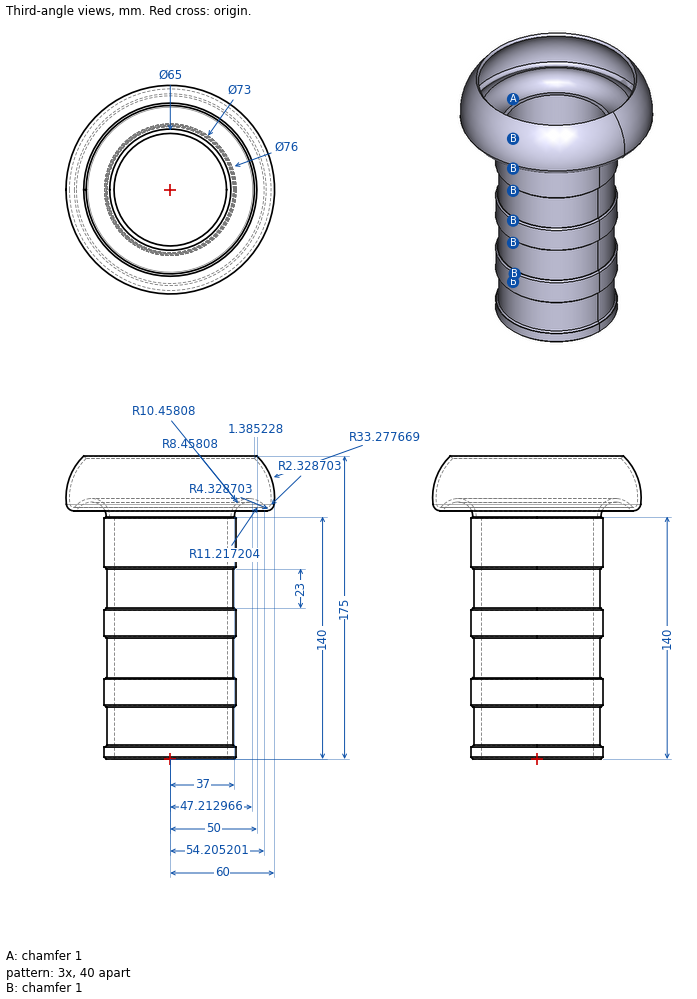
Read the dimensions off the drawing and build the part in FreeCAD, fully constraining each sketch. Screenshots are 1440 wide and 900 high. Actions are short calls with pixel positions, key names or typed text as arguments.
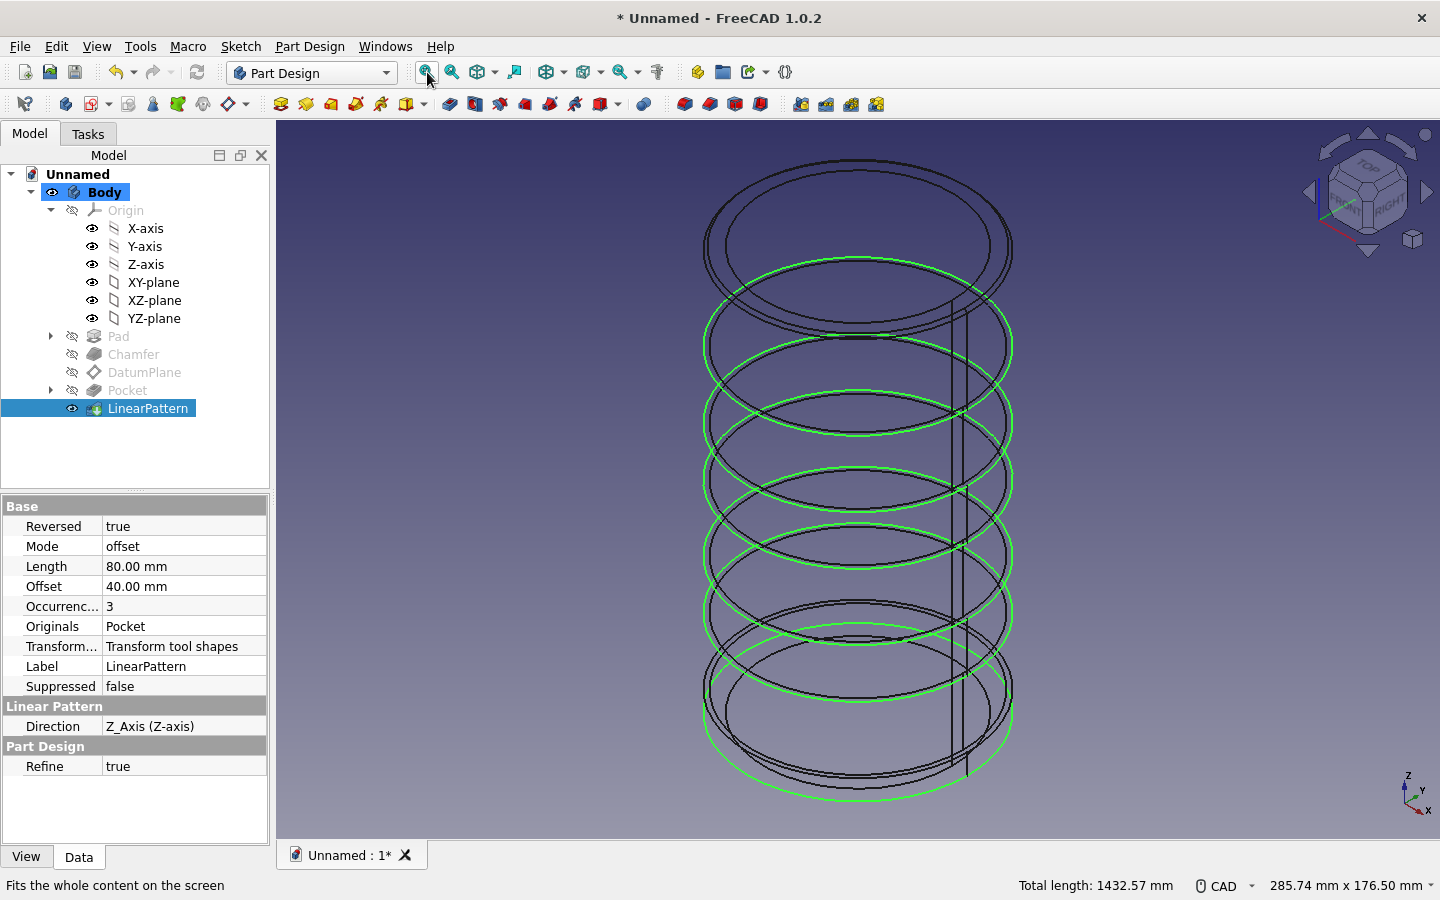
click(835, 603, ctrl)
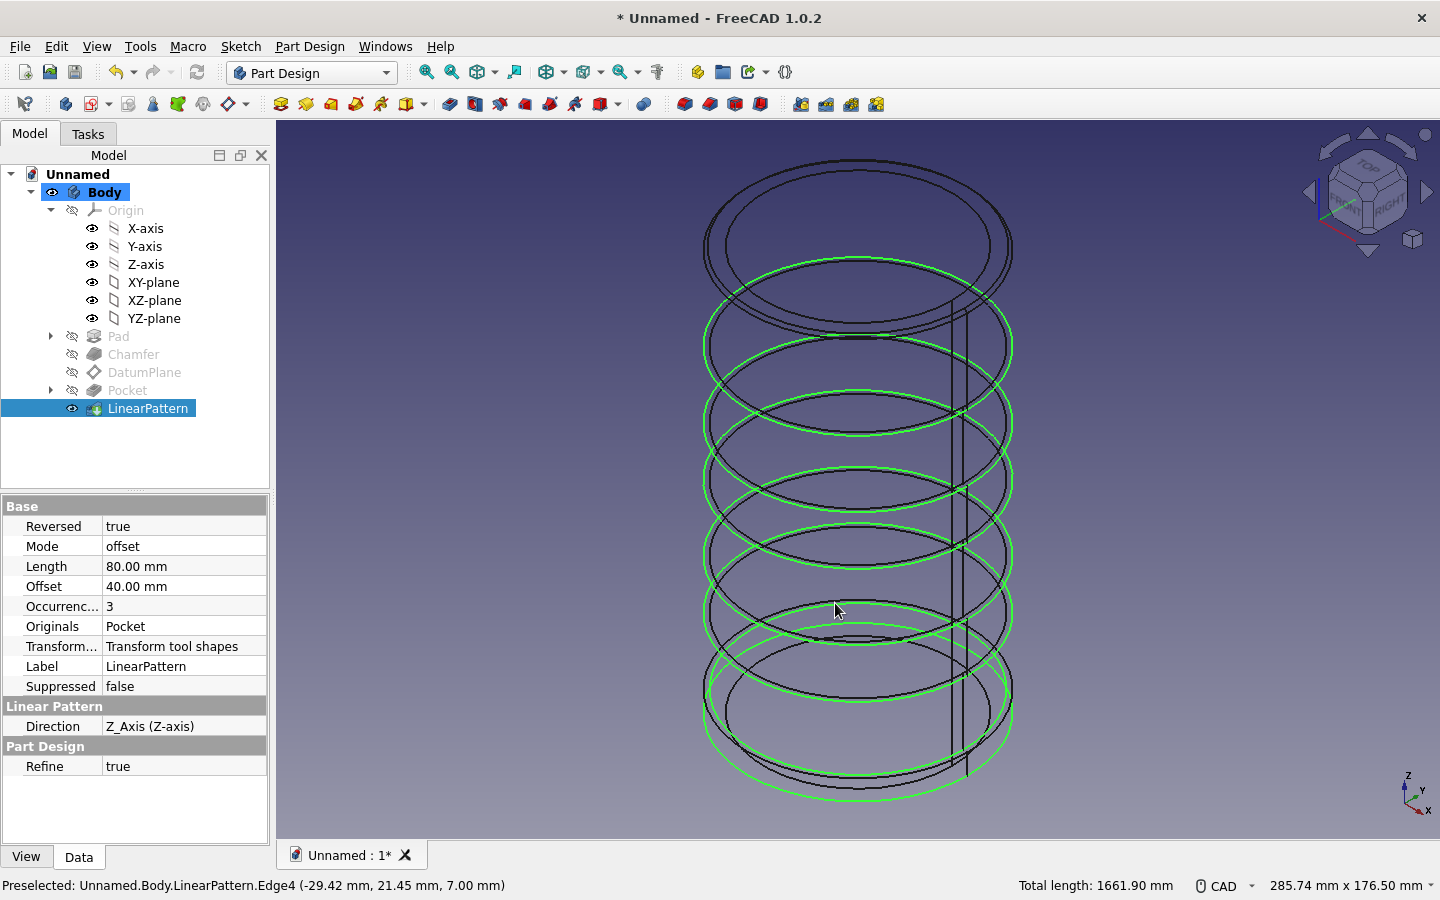
key(v)
key(1)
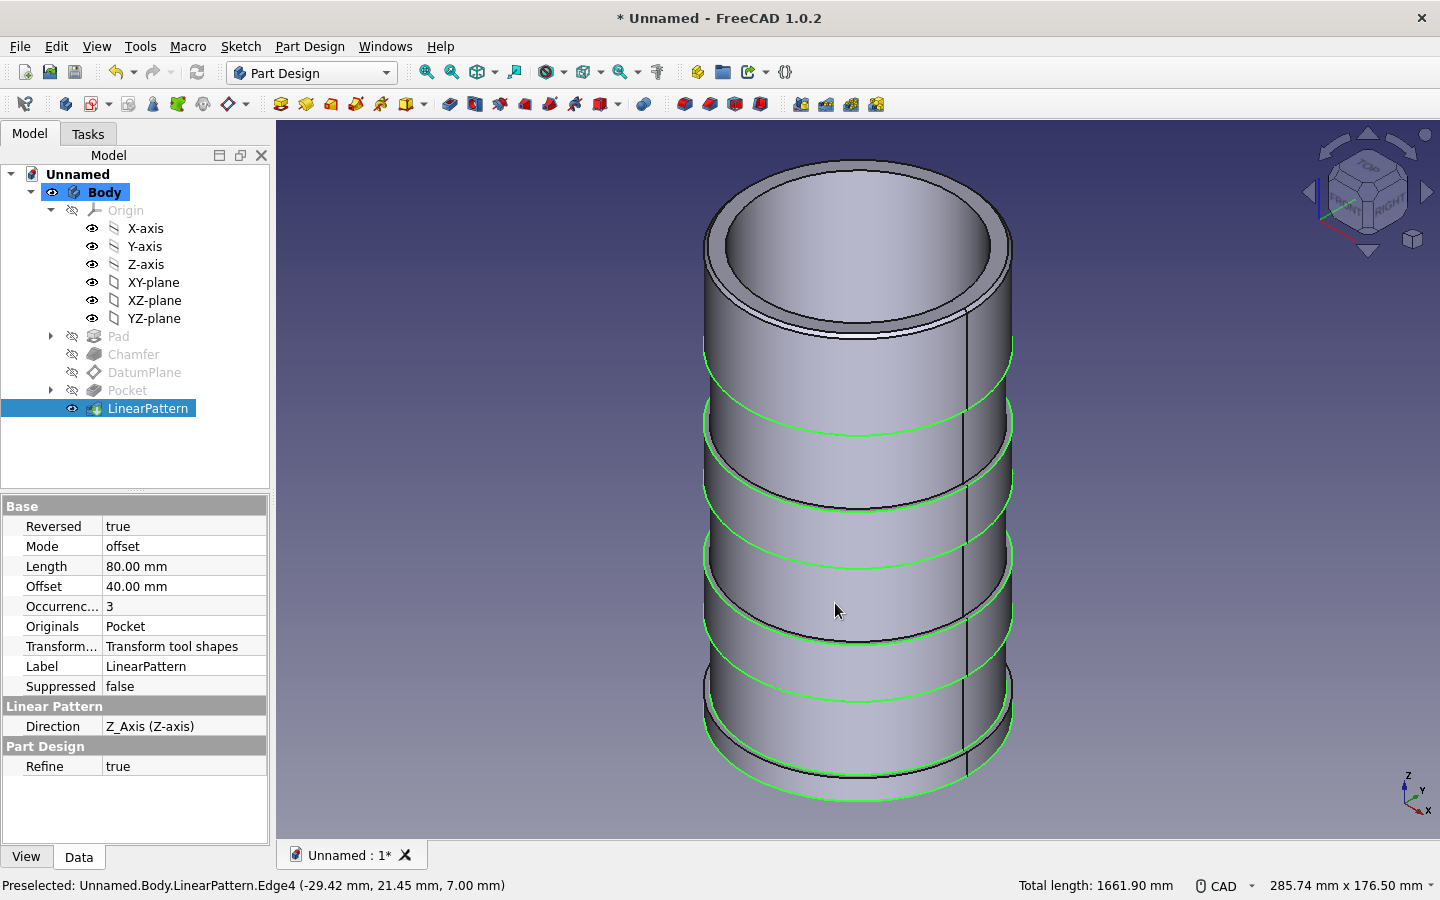
click(710, 104)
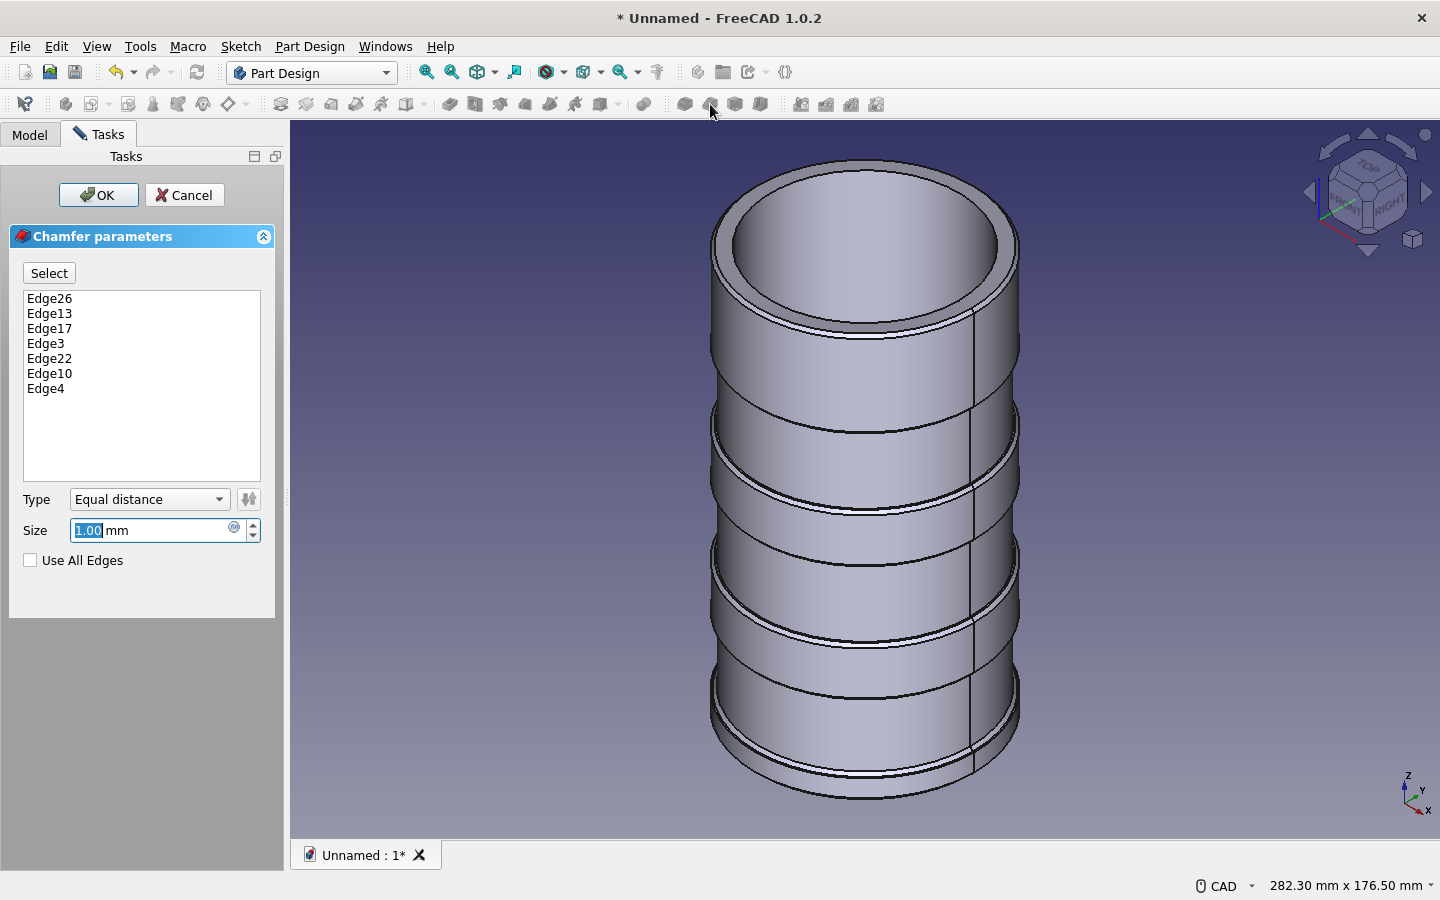
text(1)
key(Tab)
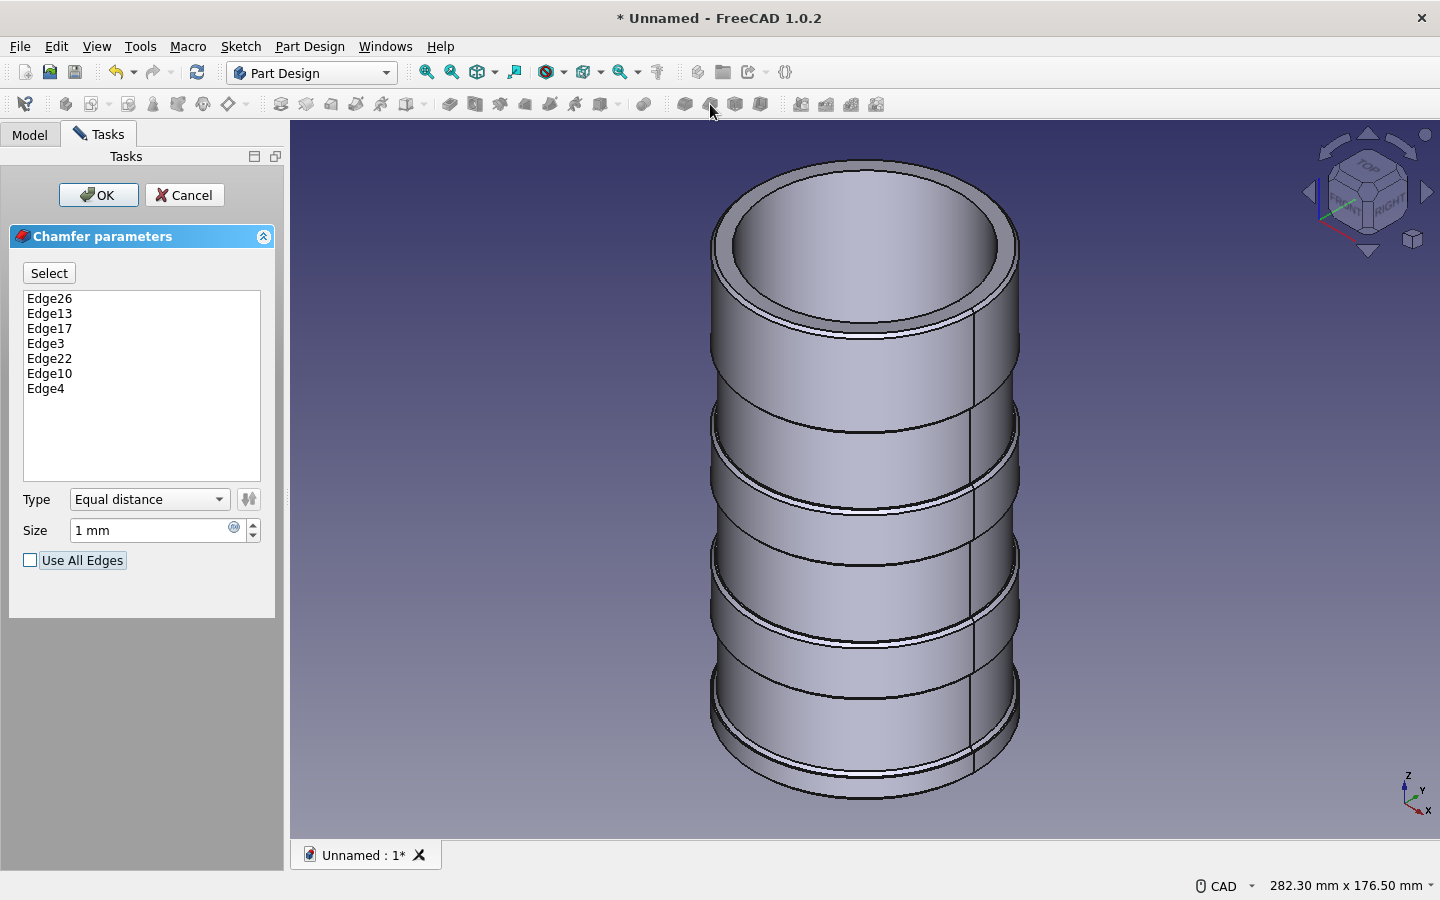
click(99, 195)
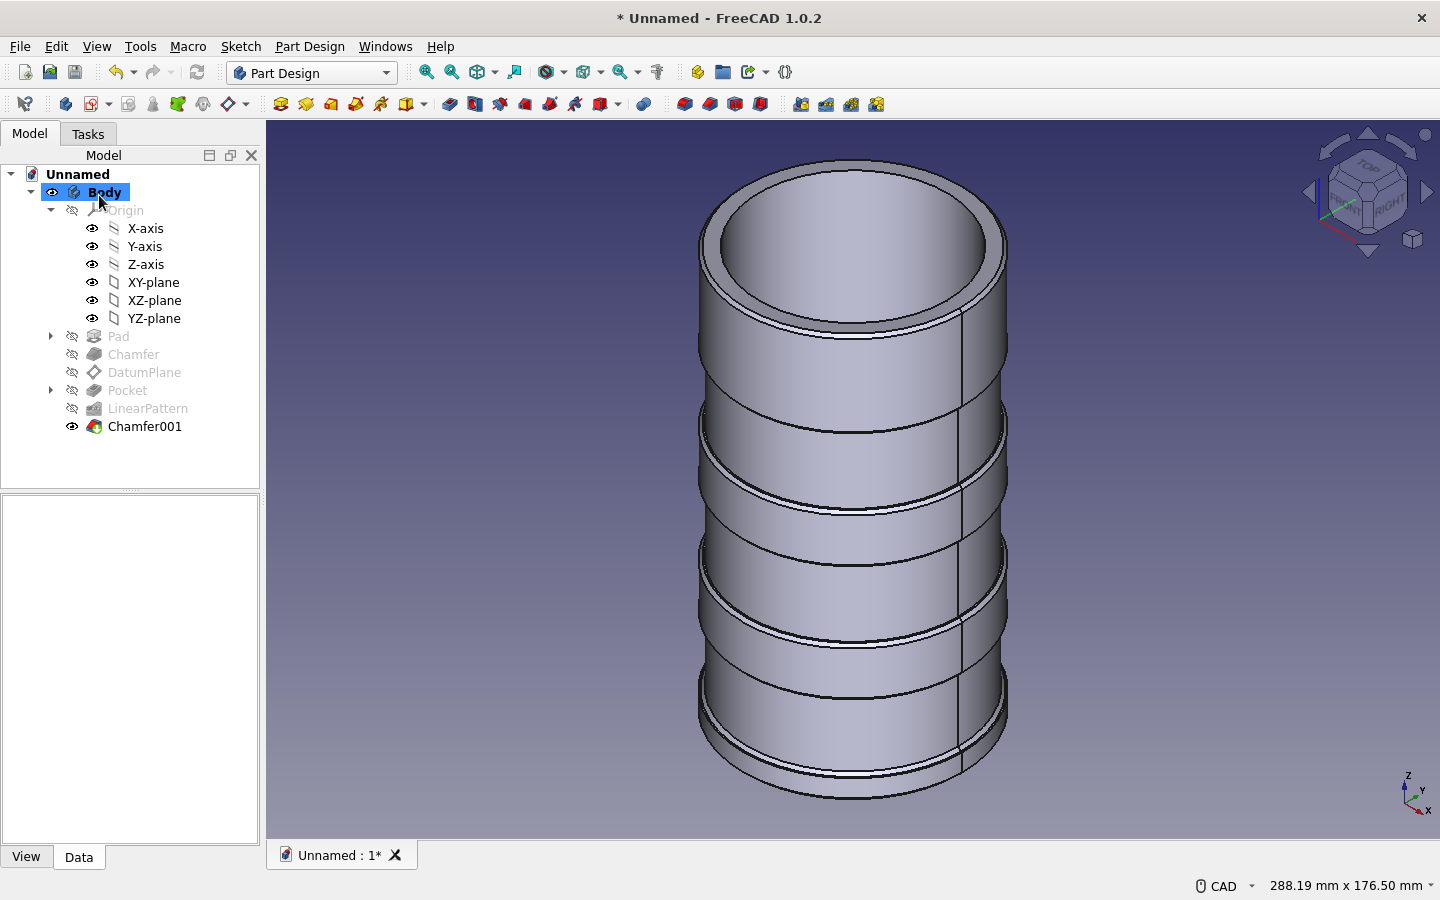
click(427, 72)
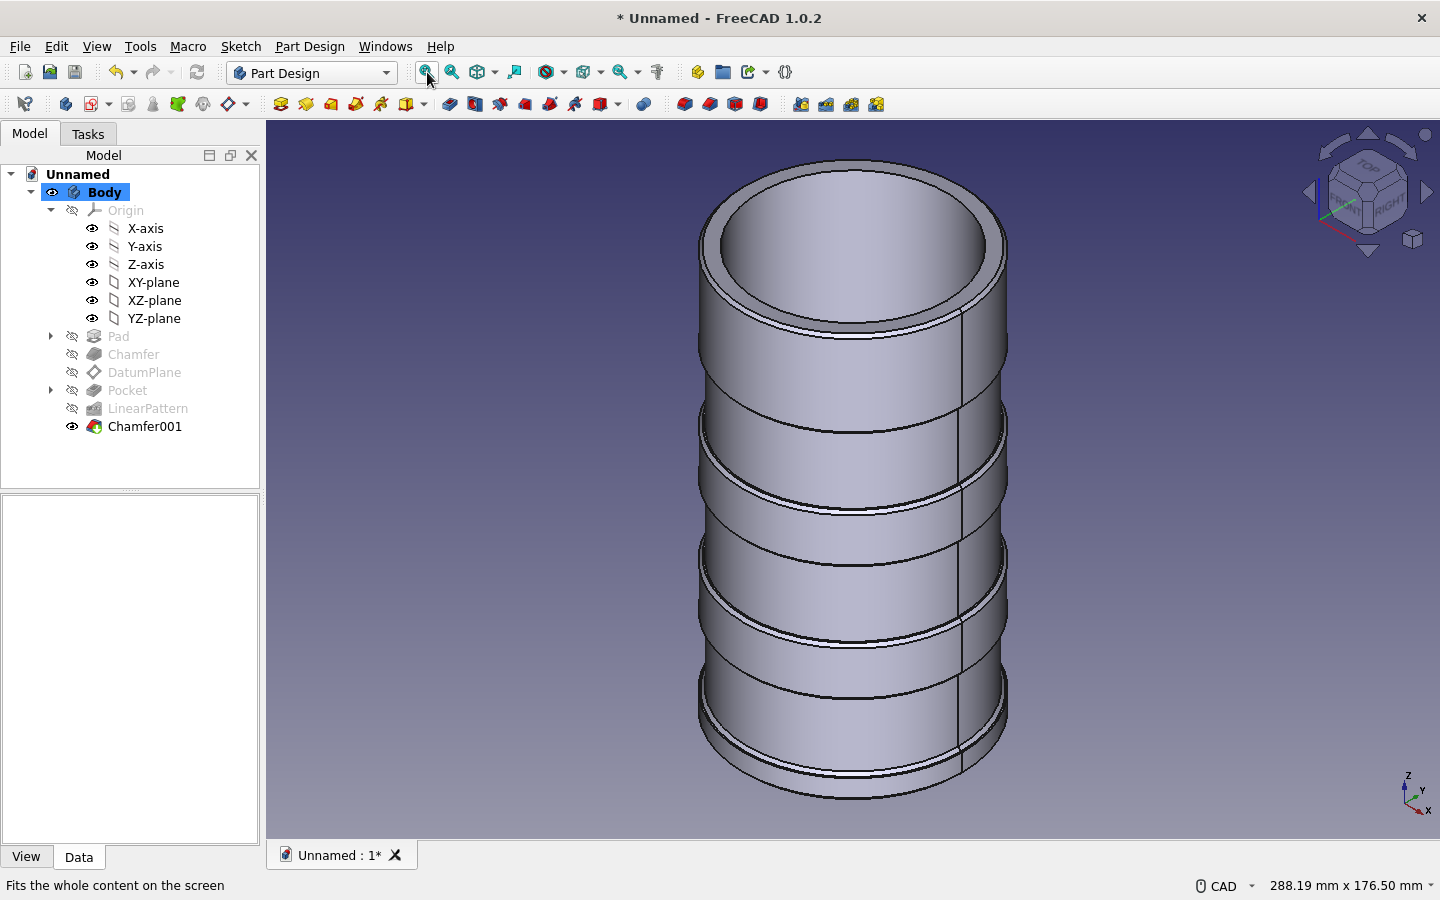
click(90, 104)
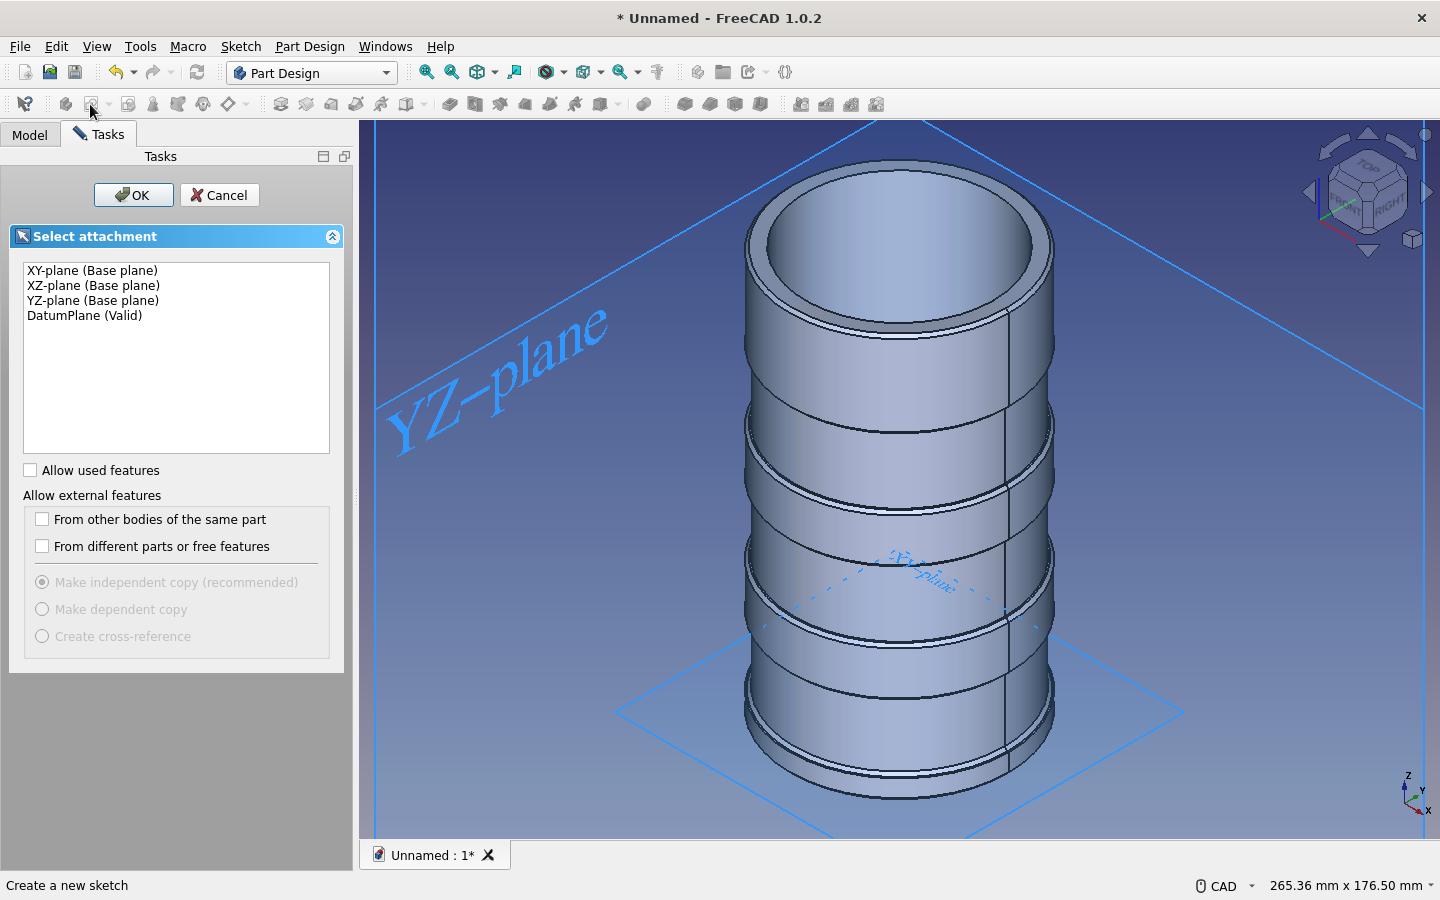
click(84, 286)